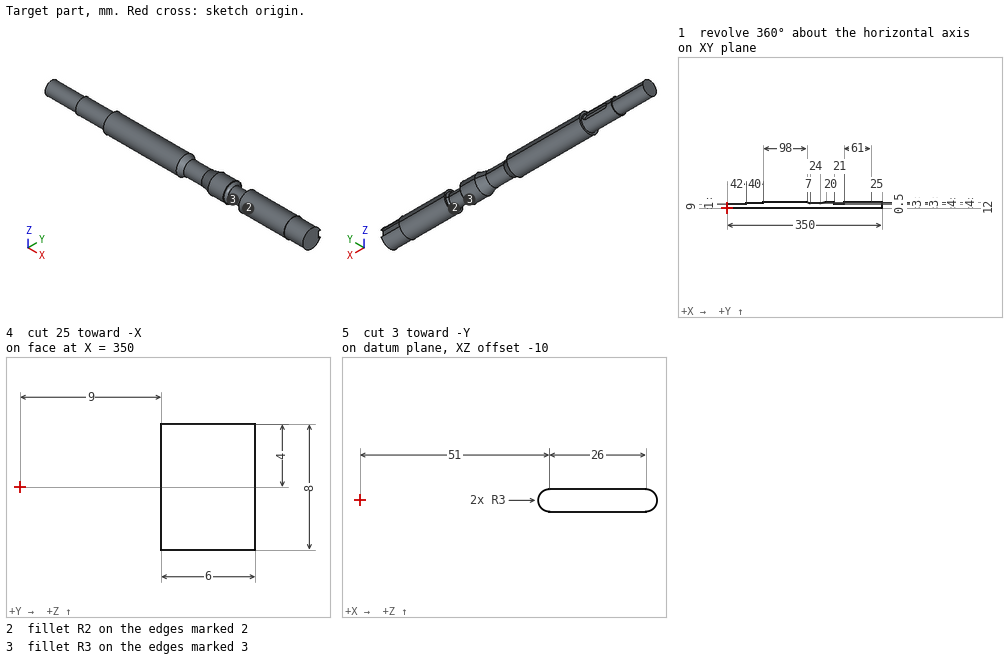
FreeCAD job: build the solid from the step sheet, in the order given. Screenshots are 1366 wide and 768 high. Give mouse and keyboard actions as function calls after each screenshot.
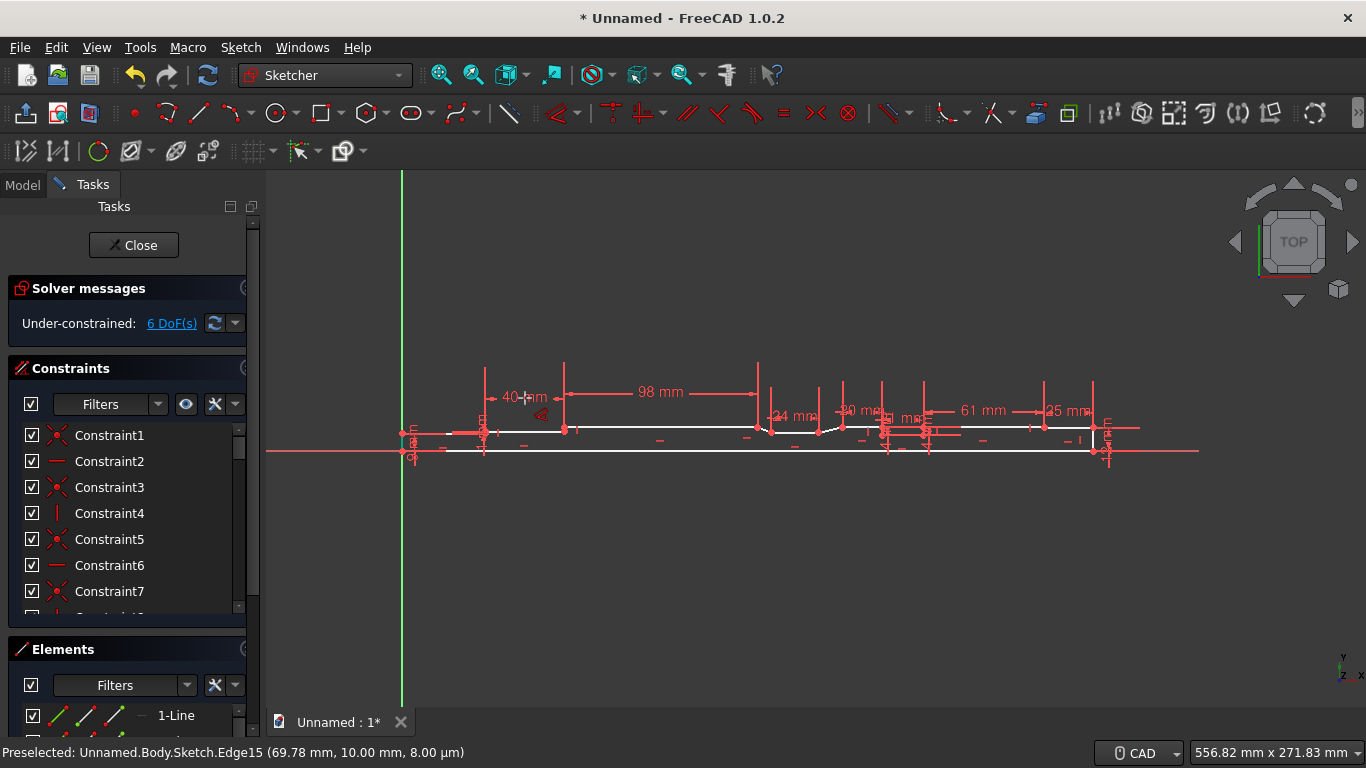
click(460, 434)
click(444, 400)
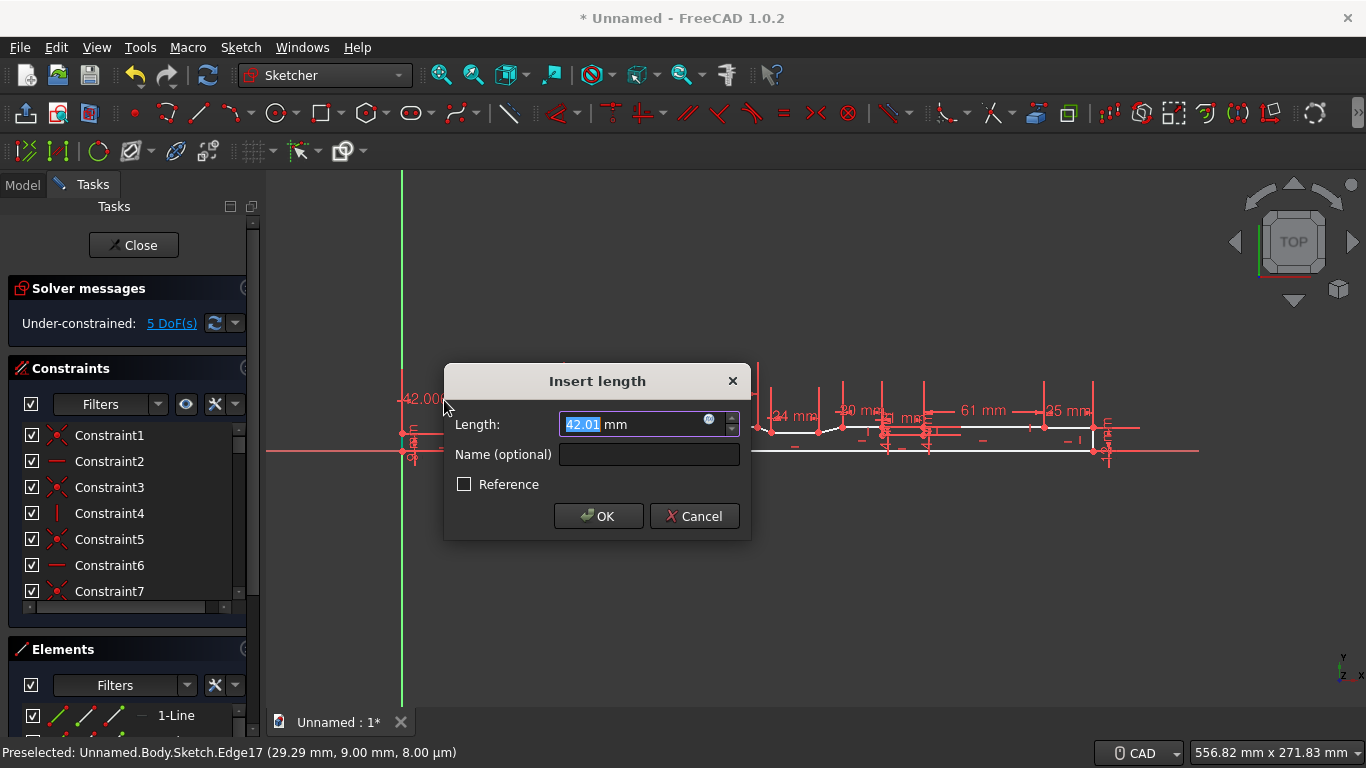
text(42)
key(Return)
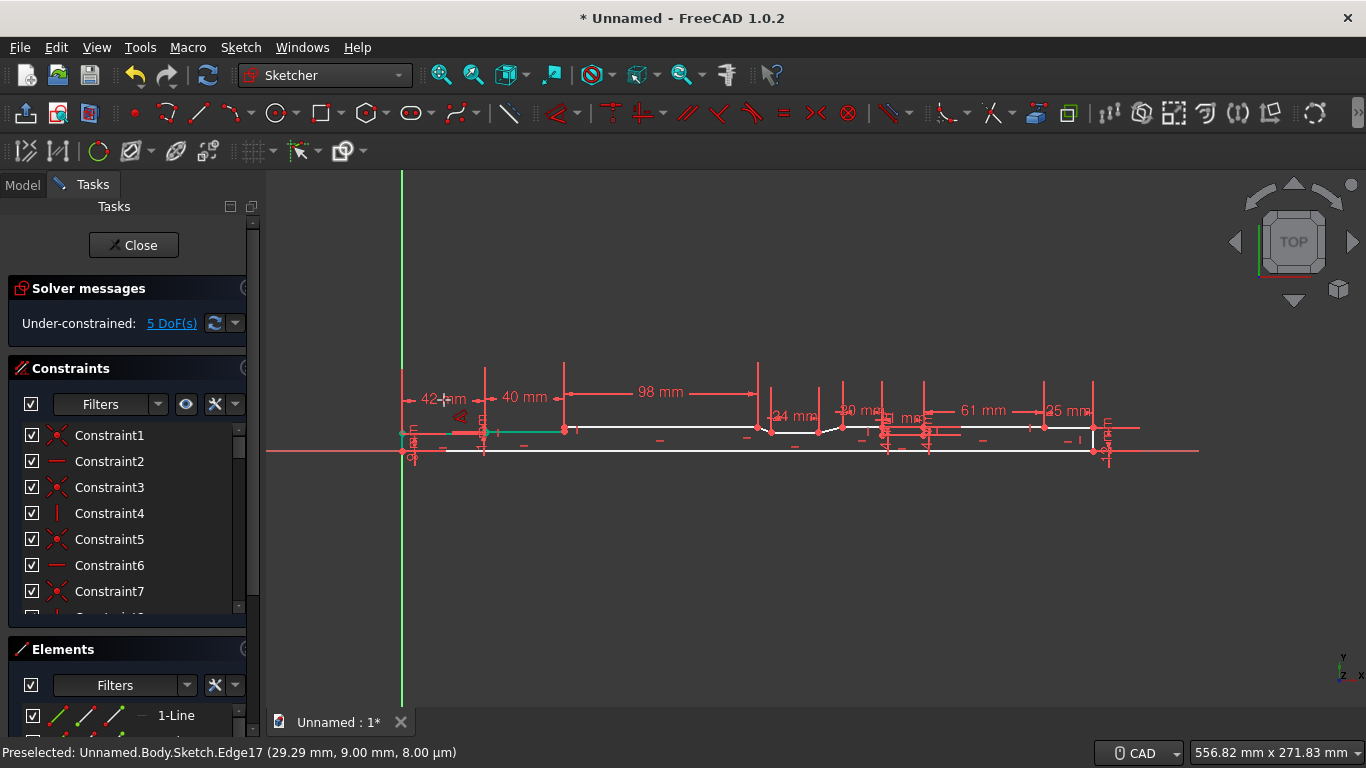
scroll(833, 429, up, 10)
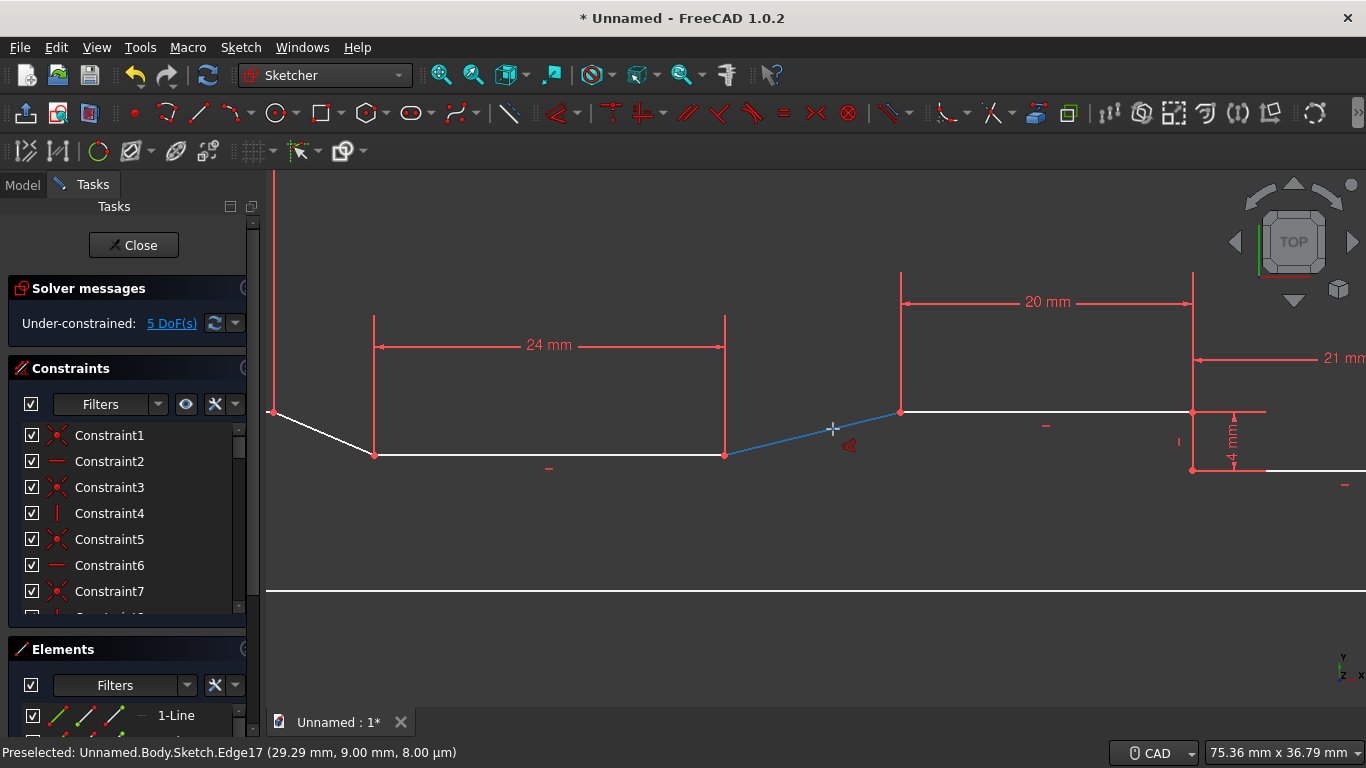
click(830, 430)
click(935, 434)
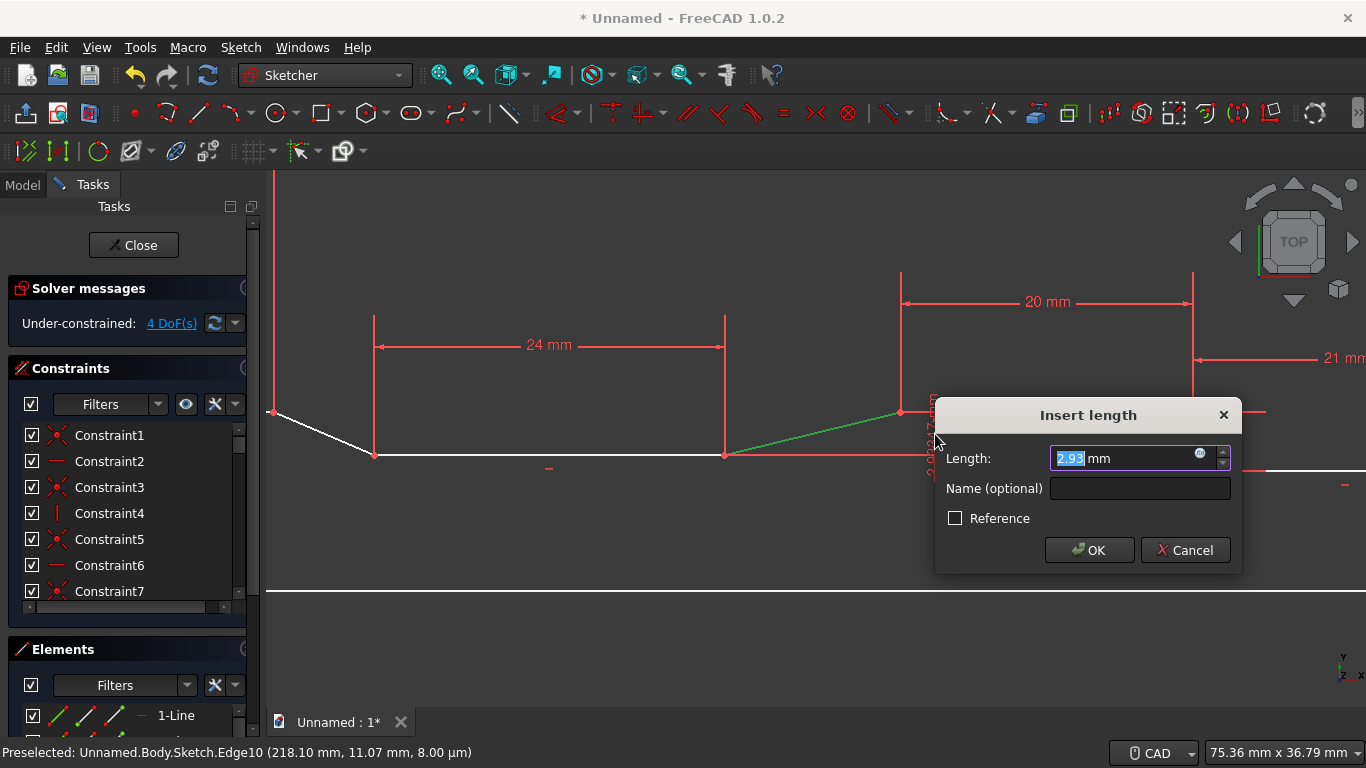
text(3)
key(Return)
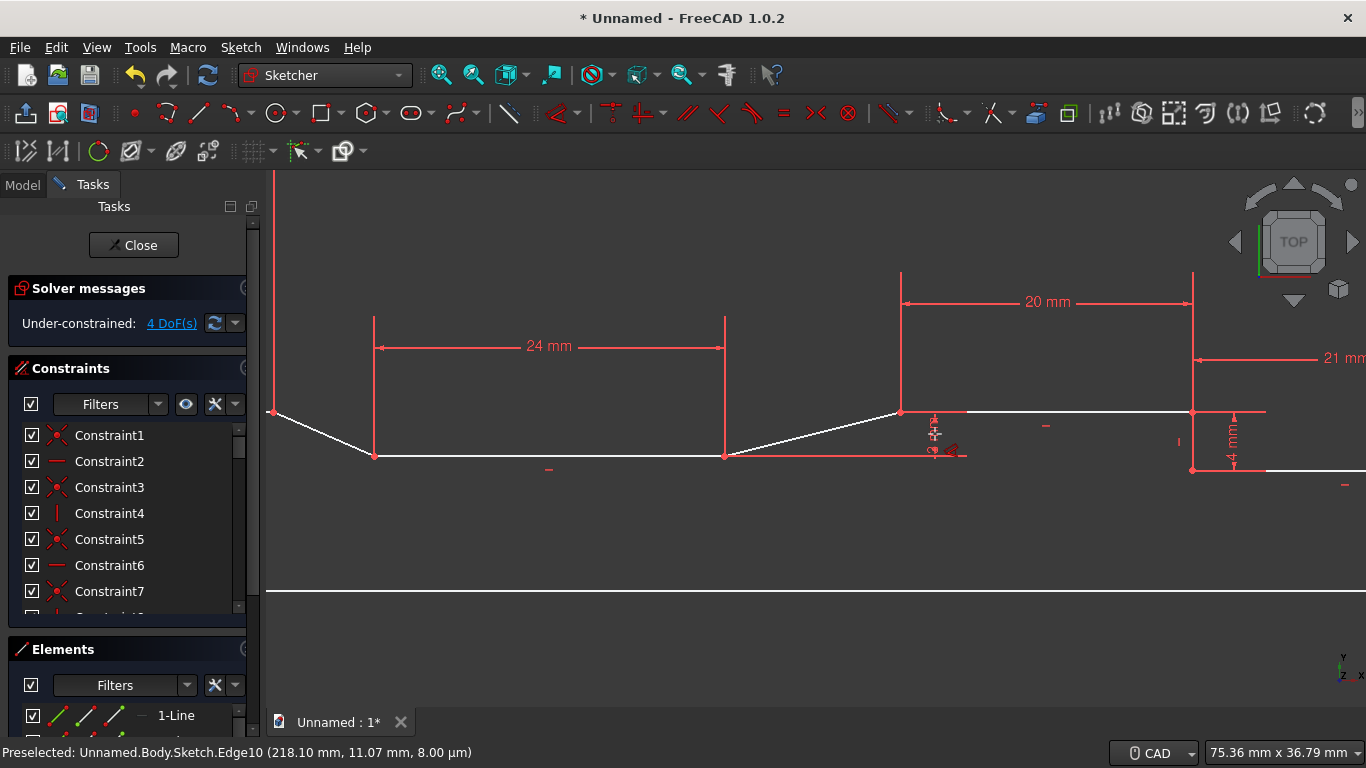
click(344, 443)
click(334, 378)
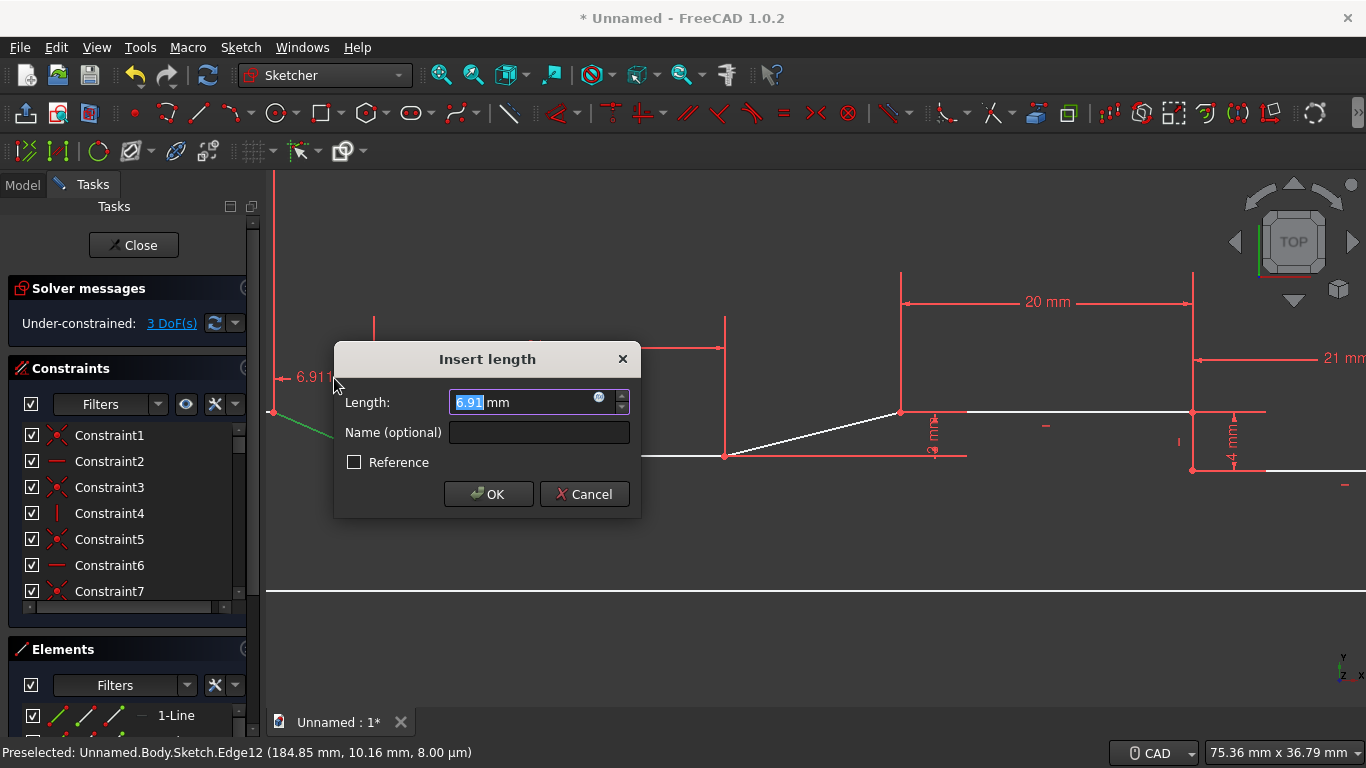
text(7)
key(Return)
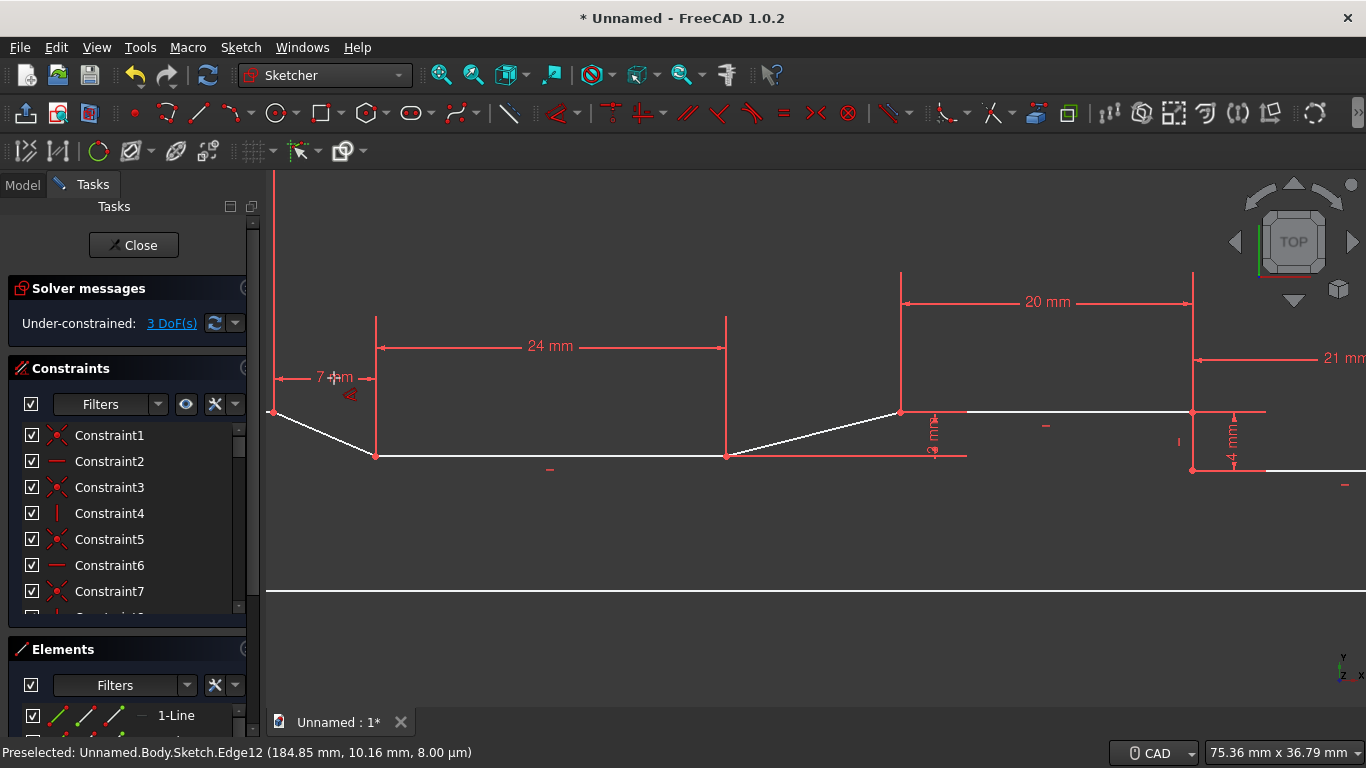
click(345, 443)
click(410, 434)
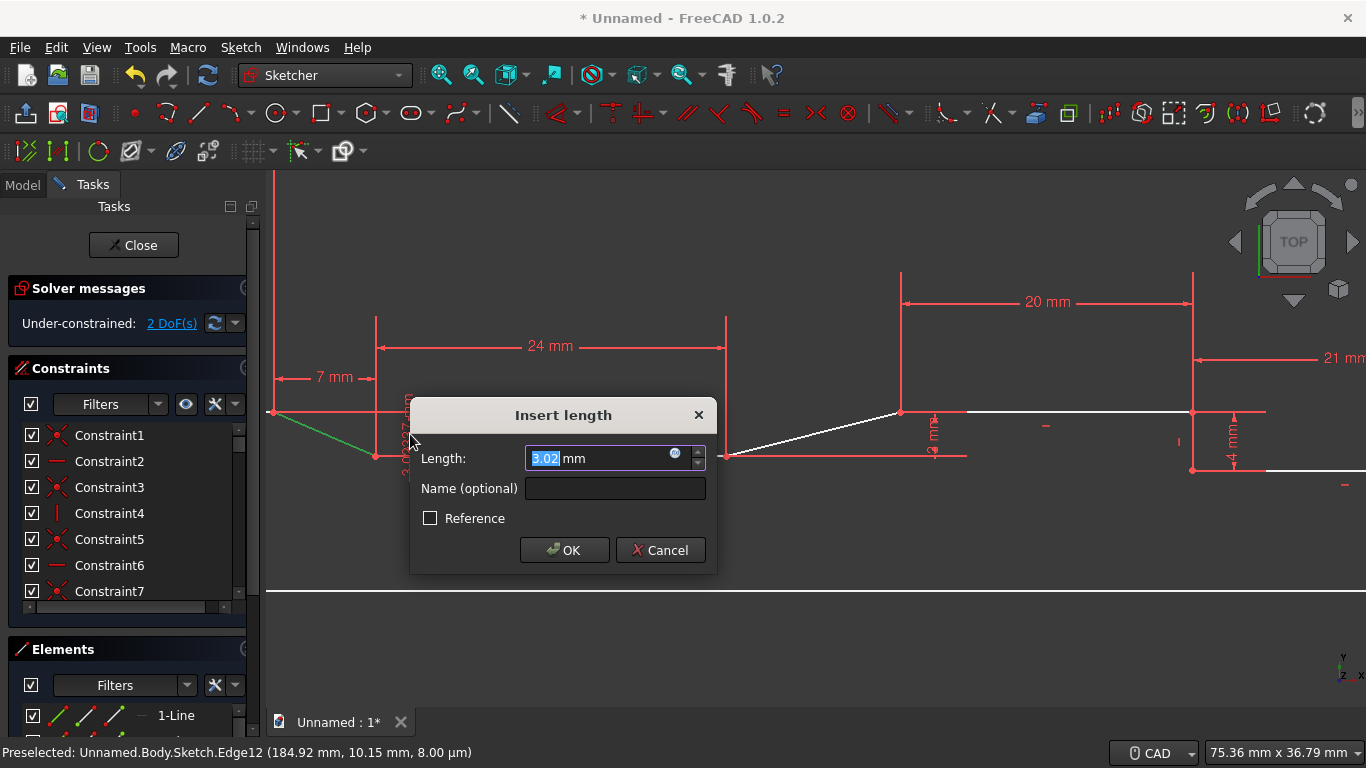
text(3)
key(Return)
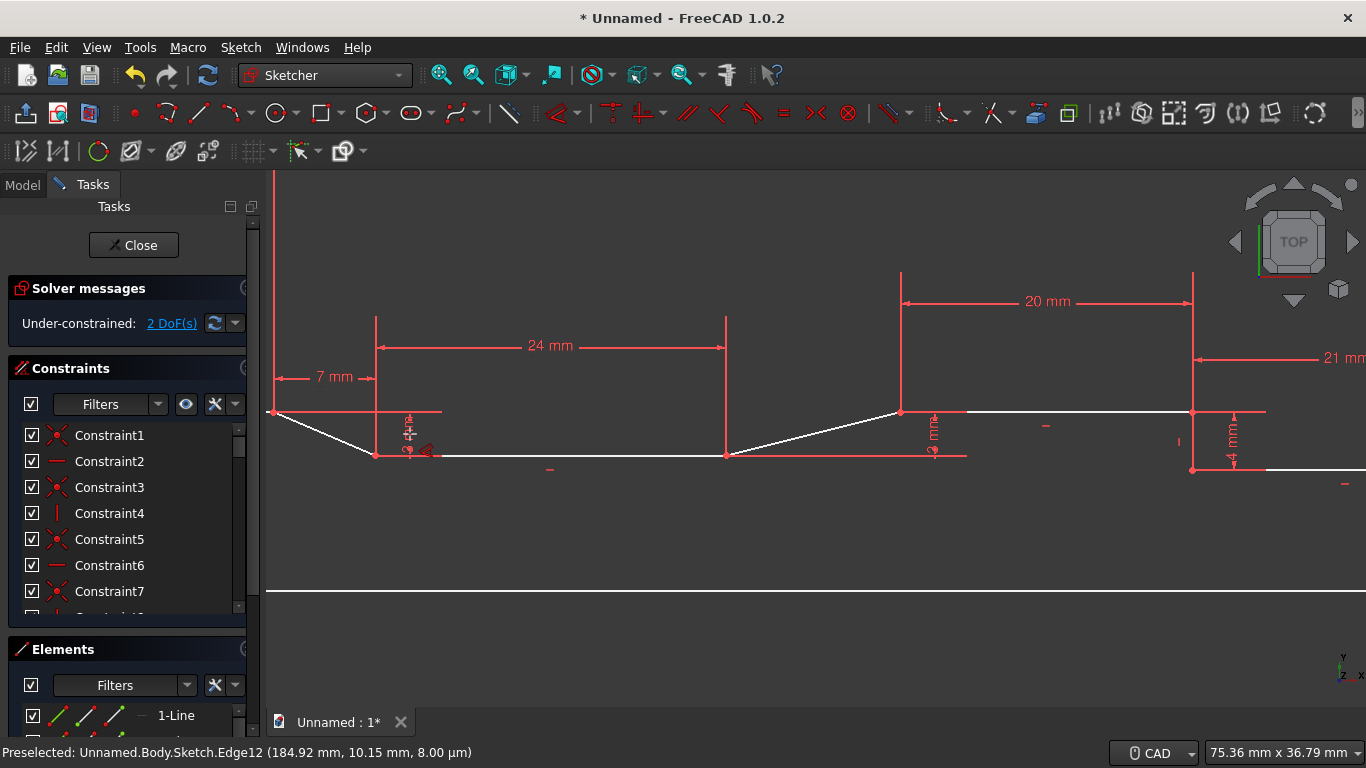
scroll(833, 429, down, 10)